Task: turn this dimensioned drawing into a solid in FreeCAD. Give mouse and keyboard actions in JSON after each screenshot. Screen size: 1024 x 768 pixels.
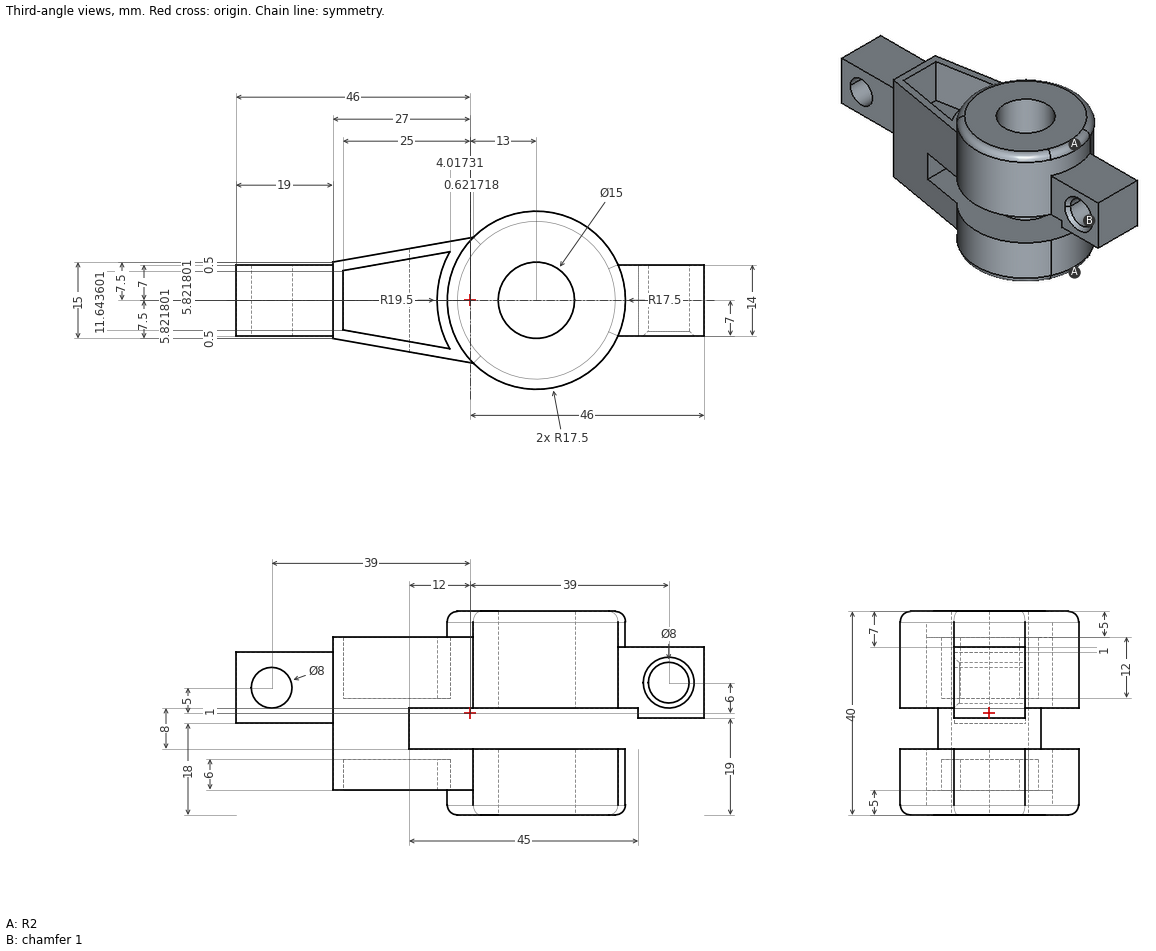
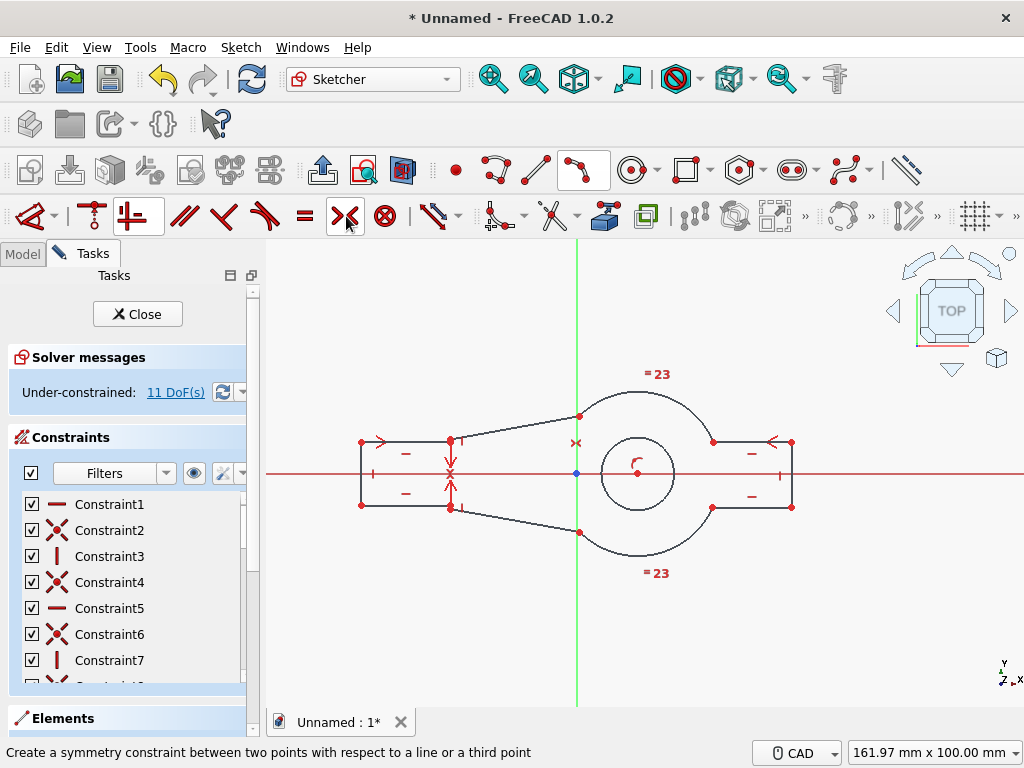
{"action": "left_click", "coordinate": [683, 405]}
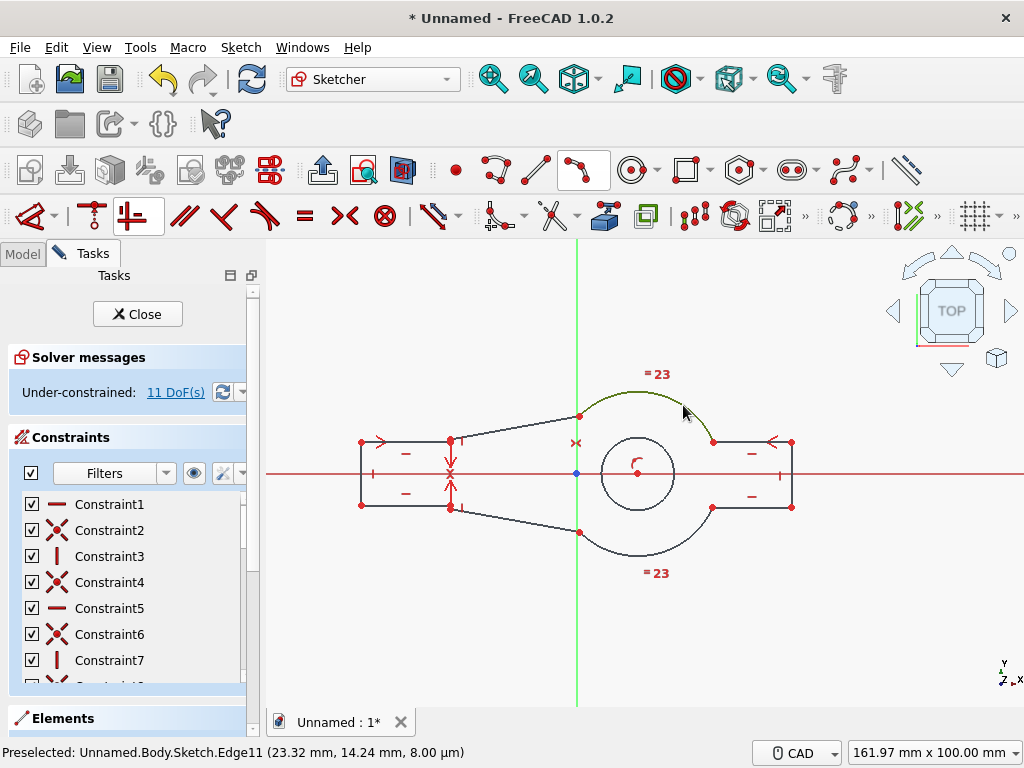
{"action": "key", "text": "k r"}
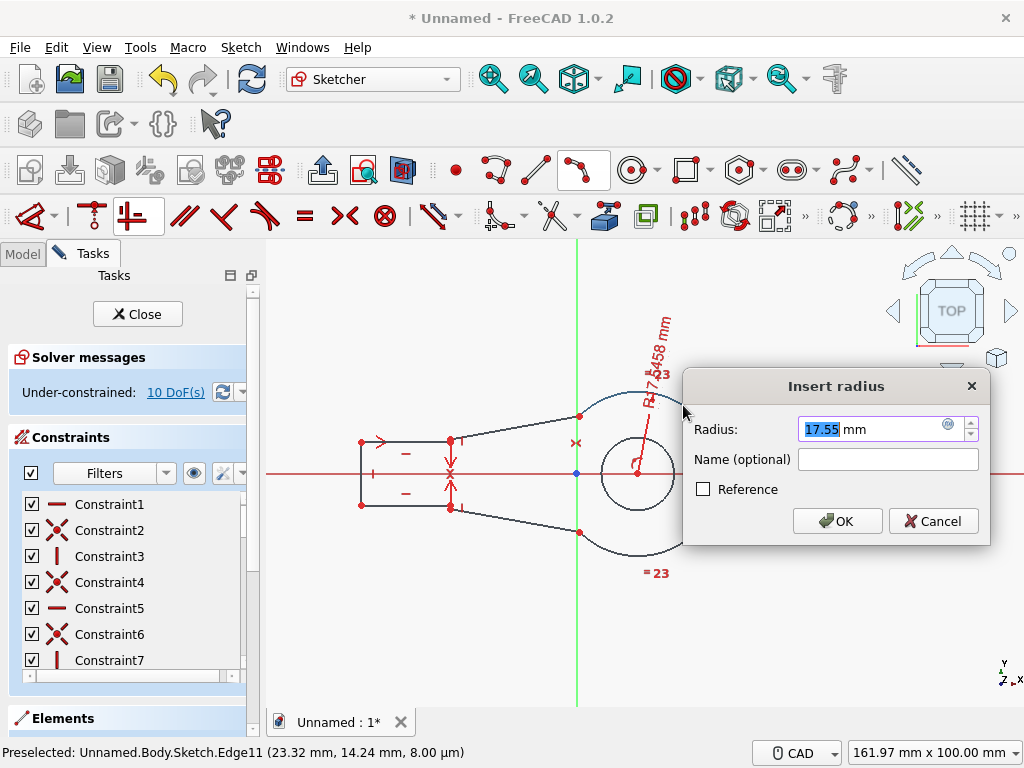
{"action": "type", "text": "17.5"}
{"action": "key", "text": "Return"}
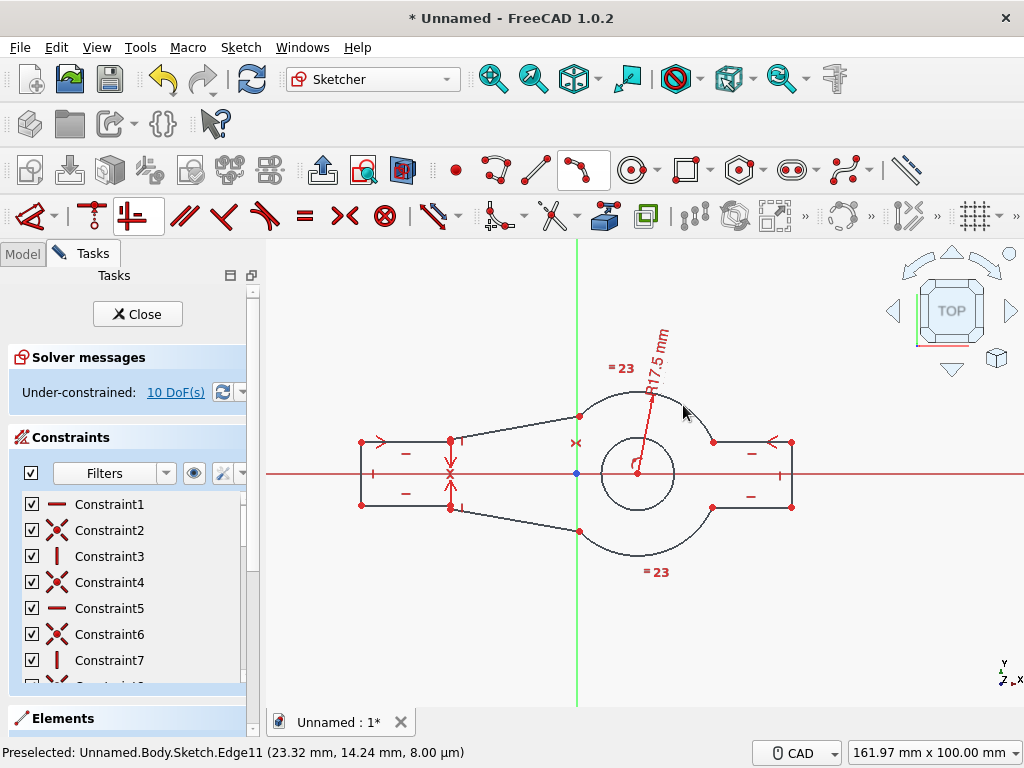
{"action": "left_click", "coordinate": [663, 448]}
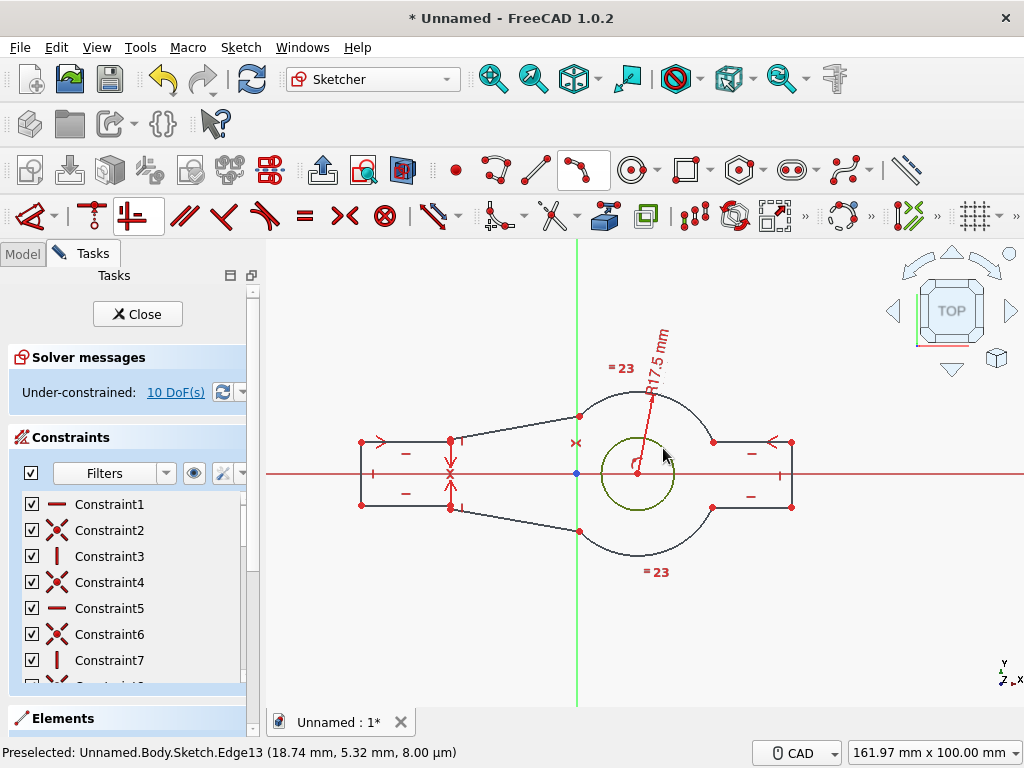
{"action": "key", "text": "k o"}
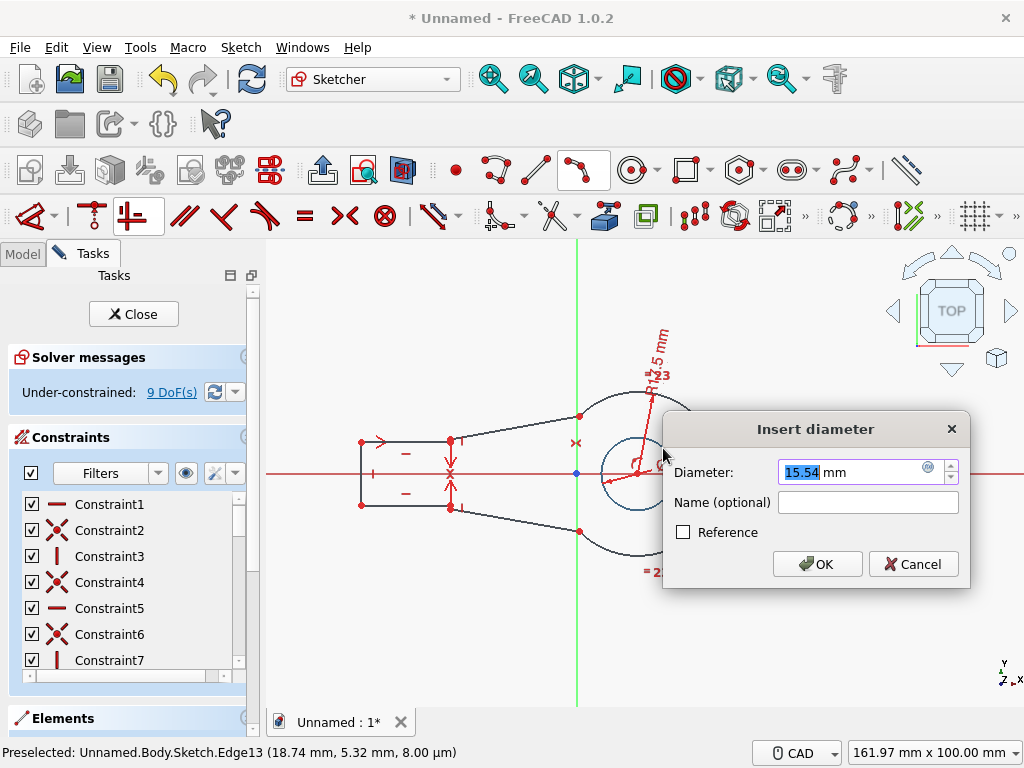
{"action": "type", "text": "15"}
{"action": "key", "text": "Return"}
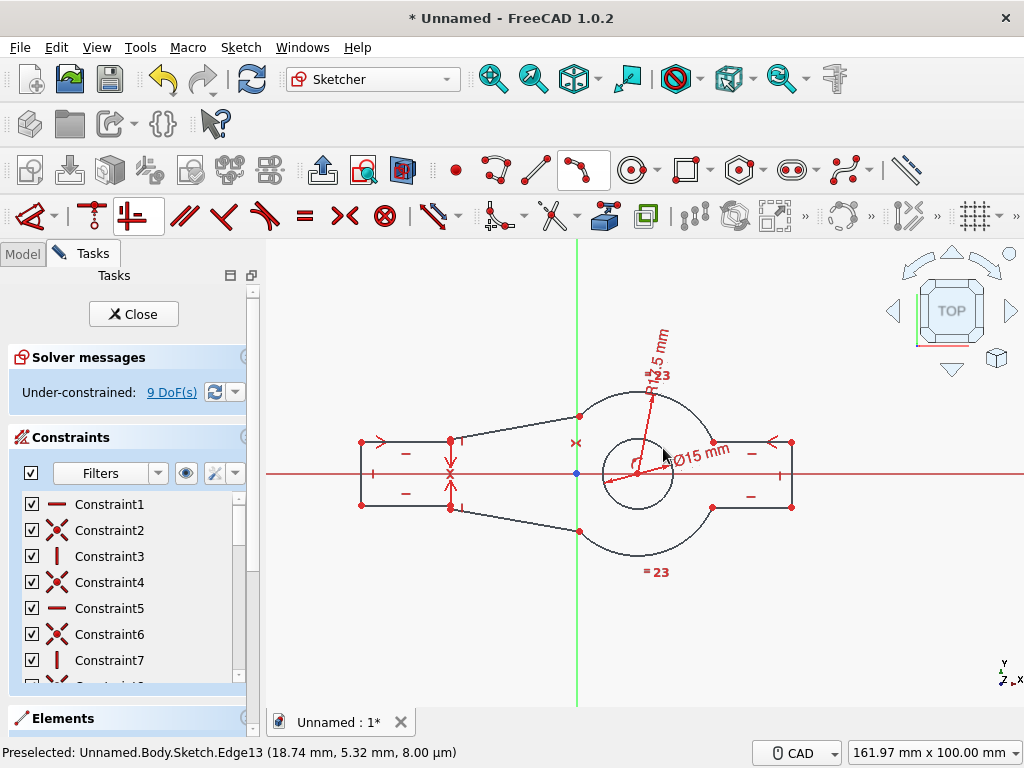
{"action": "left_click", "coordinate": [792, 488]}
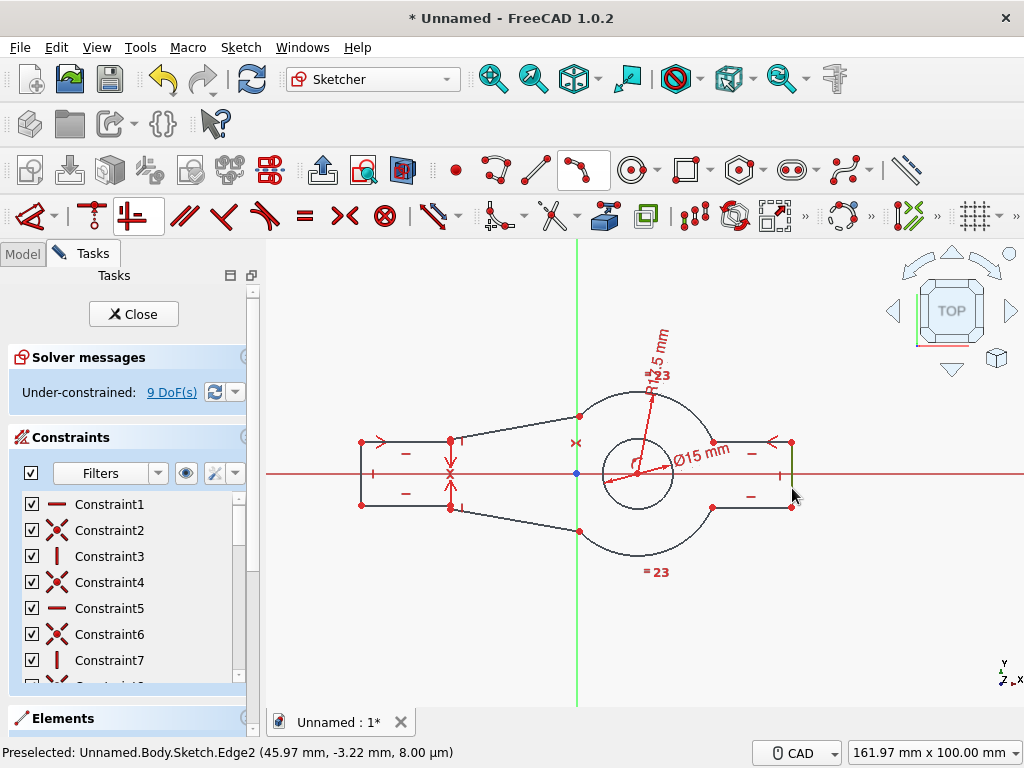
{"action": "left_click", "coordinate": [56, 216]}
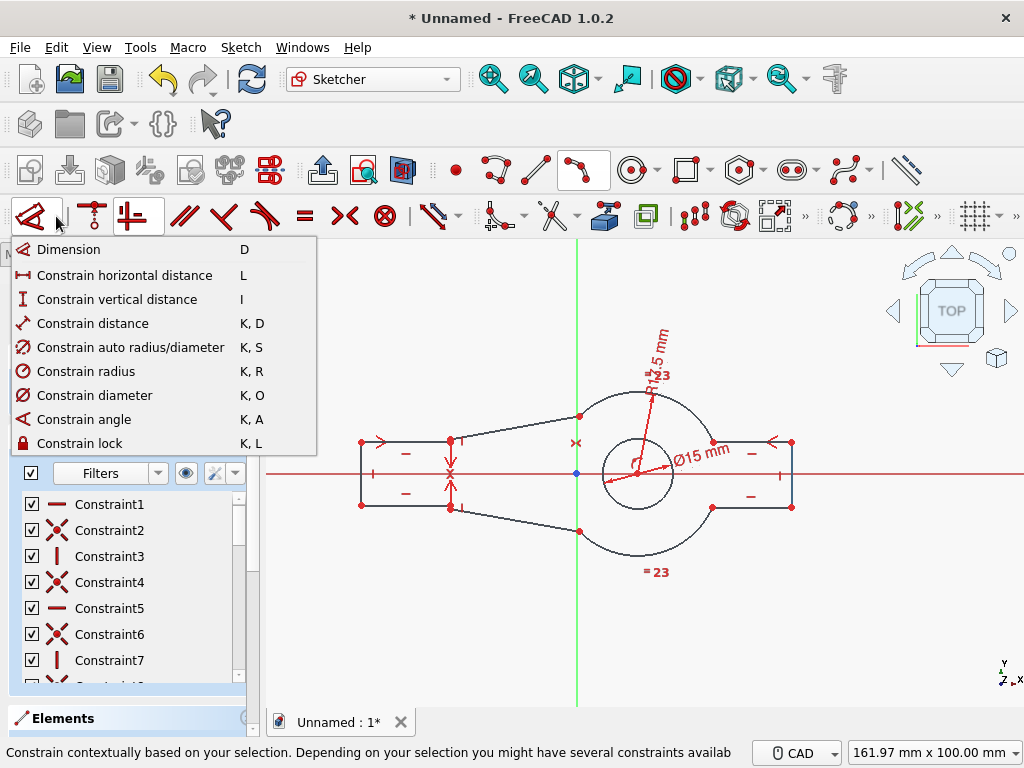
{"action": "left_click", "coordinate": [164, 299]}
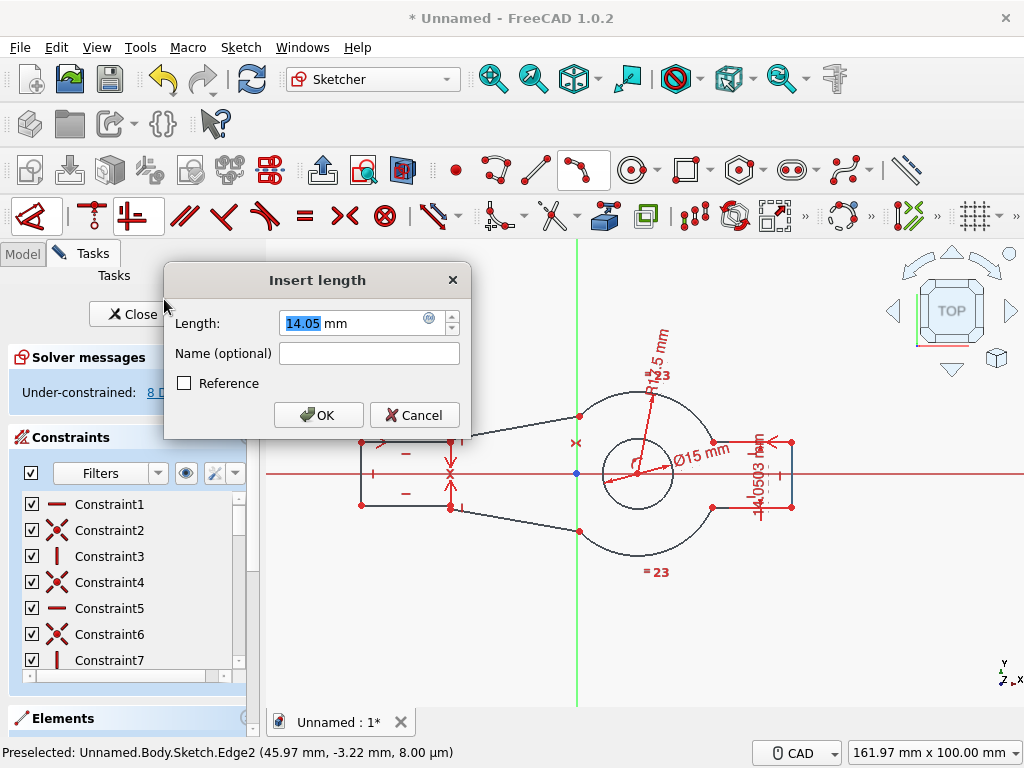
{"action": "type", "text": "14"}
{"action": "key", "text": "Return"}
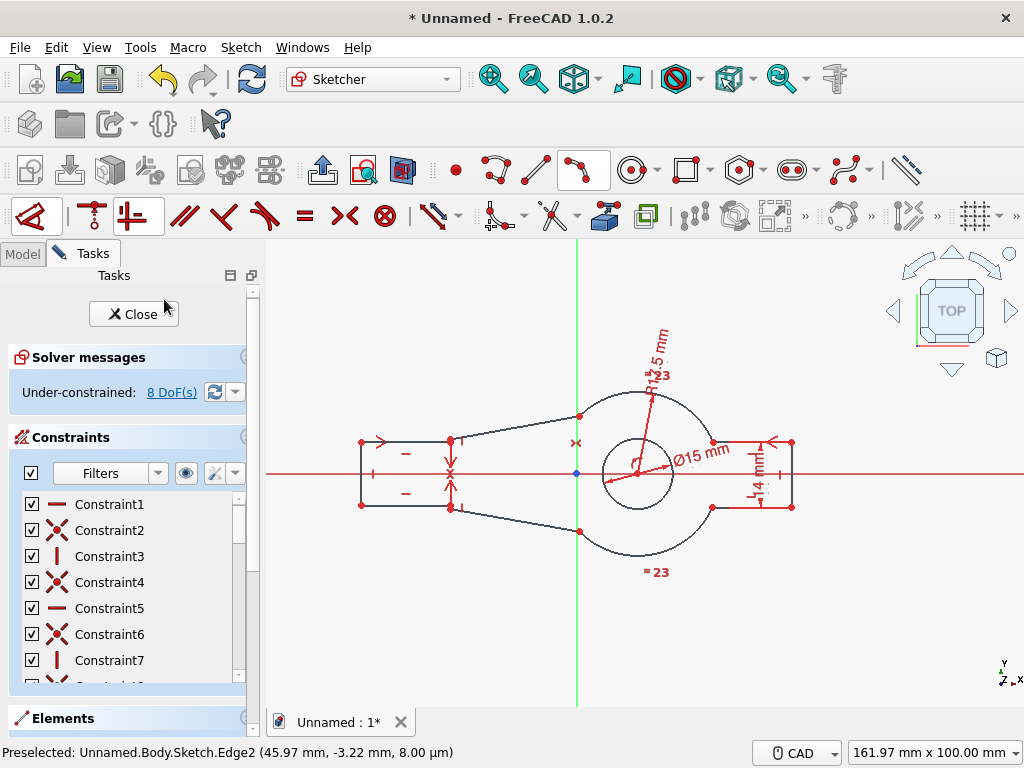
{"action": "left_click", "coordinate": [424, 442]}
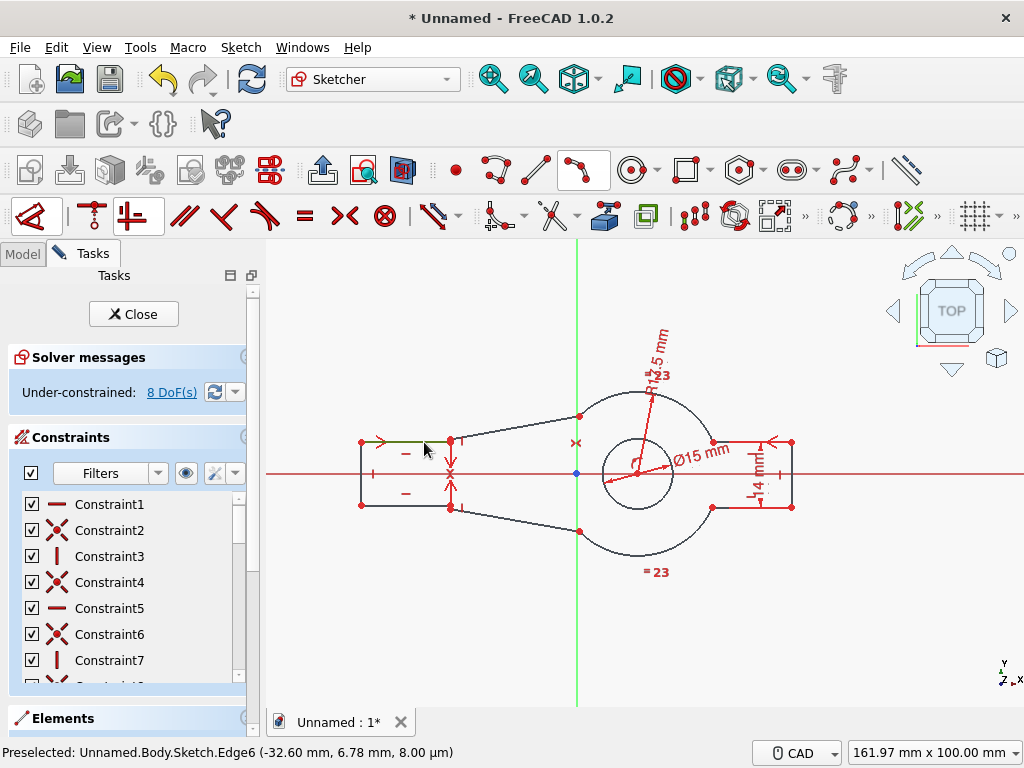
{"action": "left_click", "coordinate": [56, 216]}